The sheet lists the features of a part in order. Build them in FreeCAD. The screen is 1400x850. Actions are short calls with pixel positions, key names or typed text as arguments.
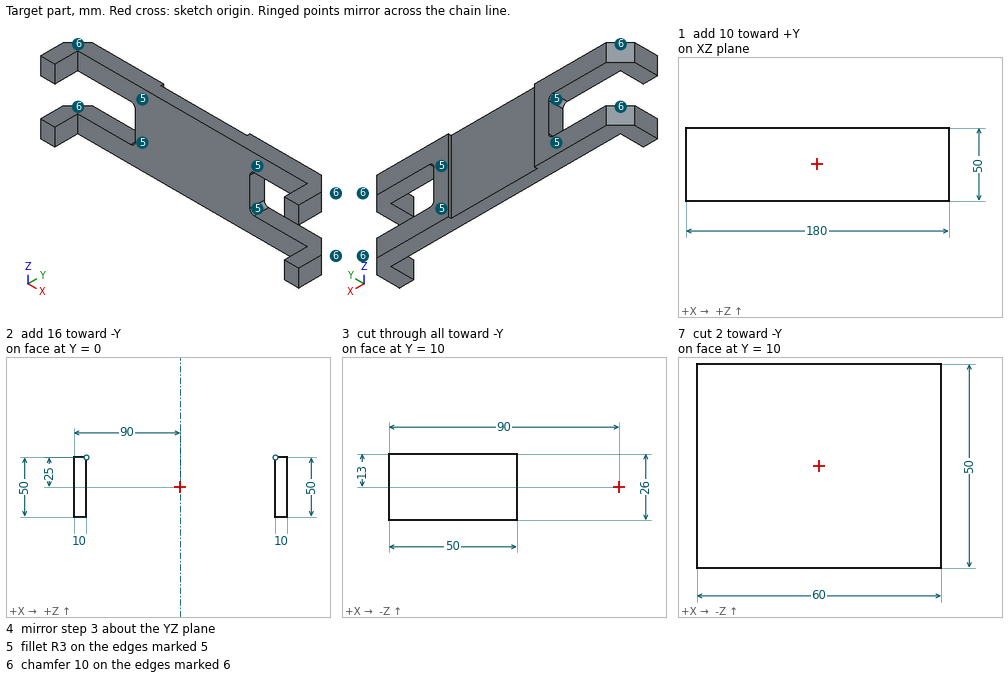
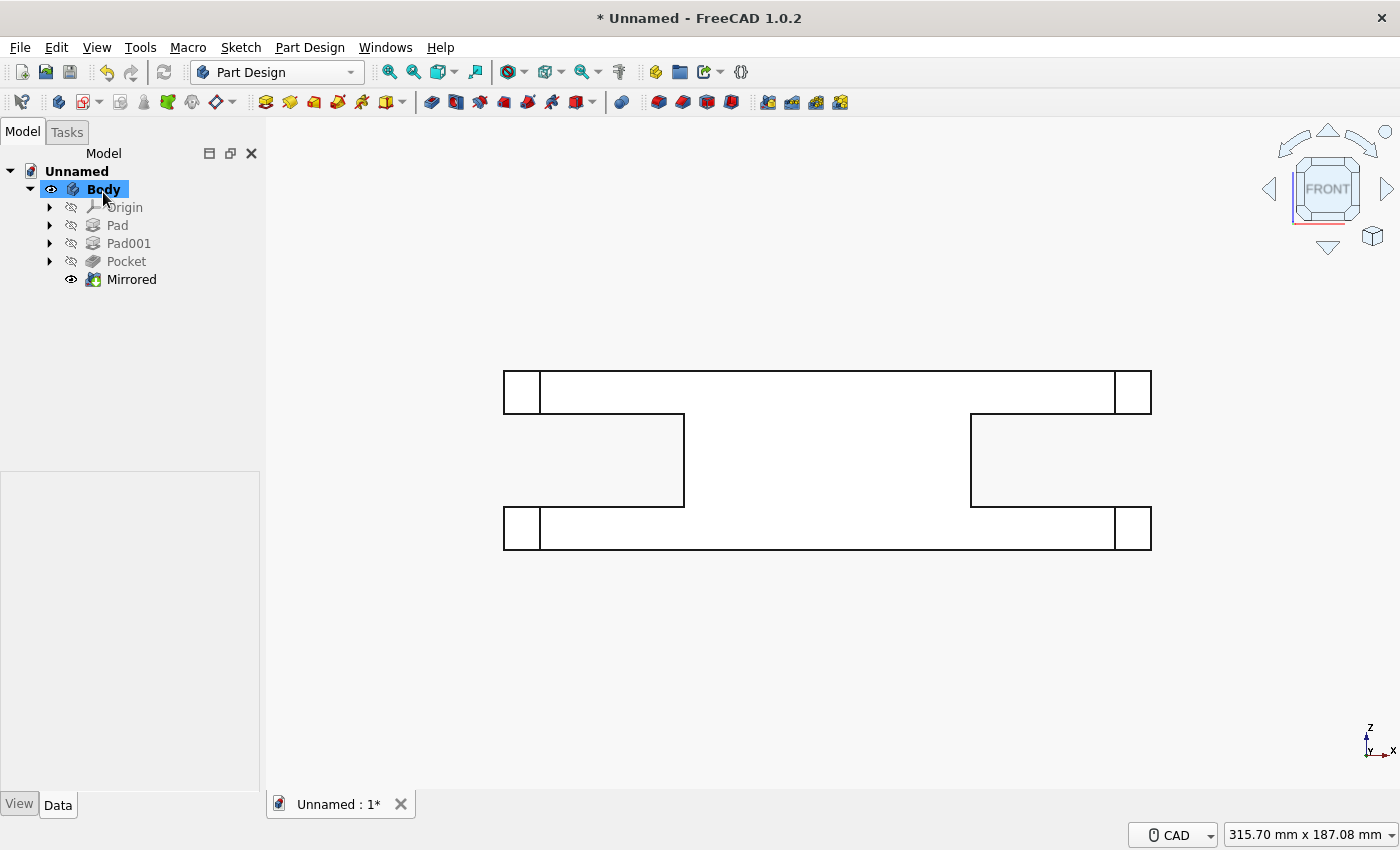
key(3)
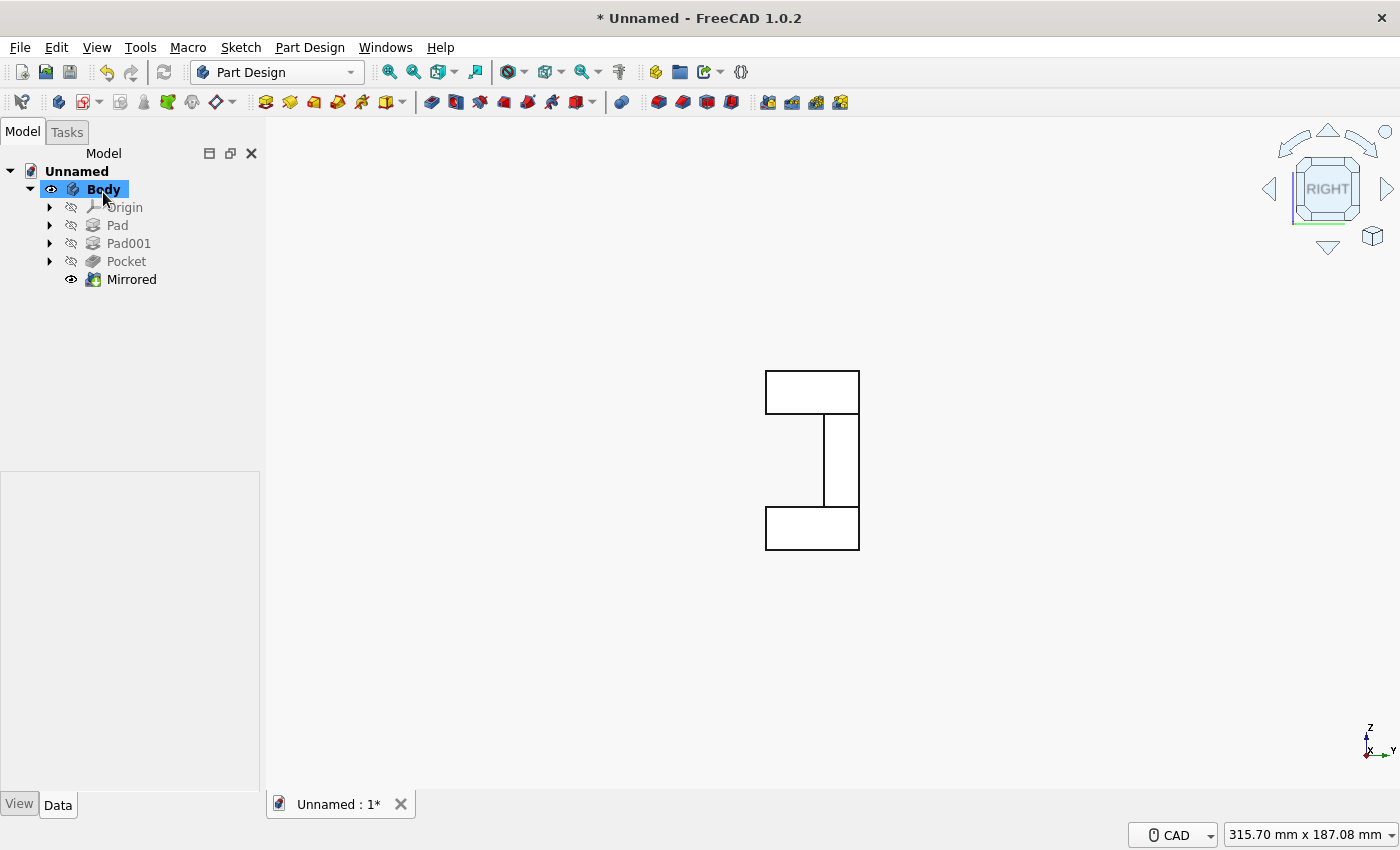
click(390, 72)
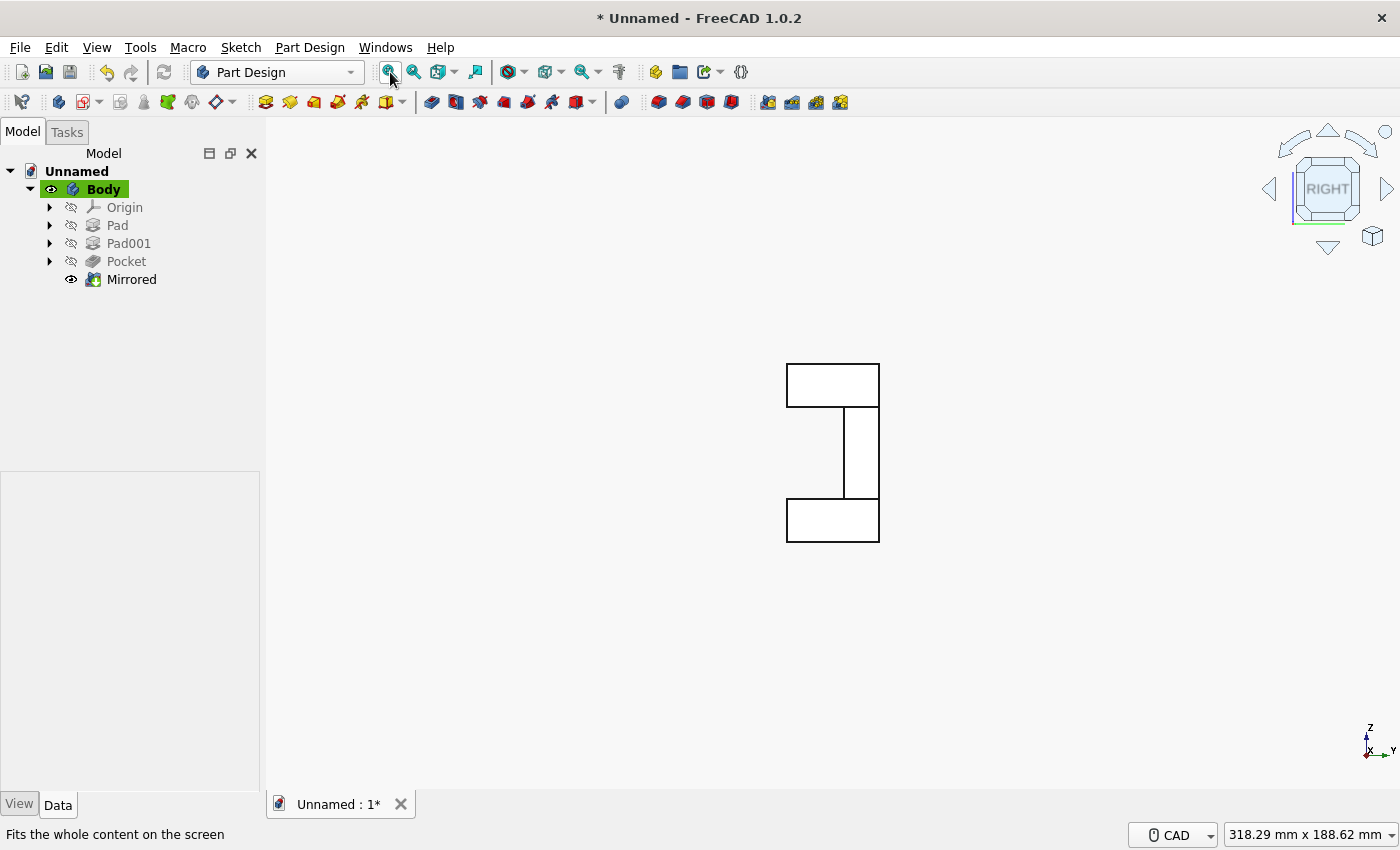
key(5)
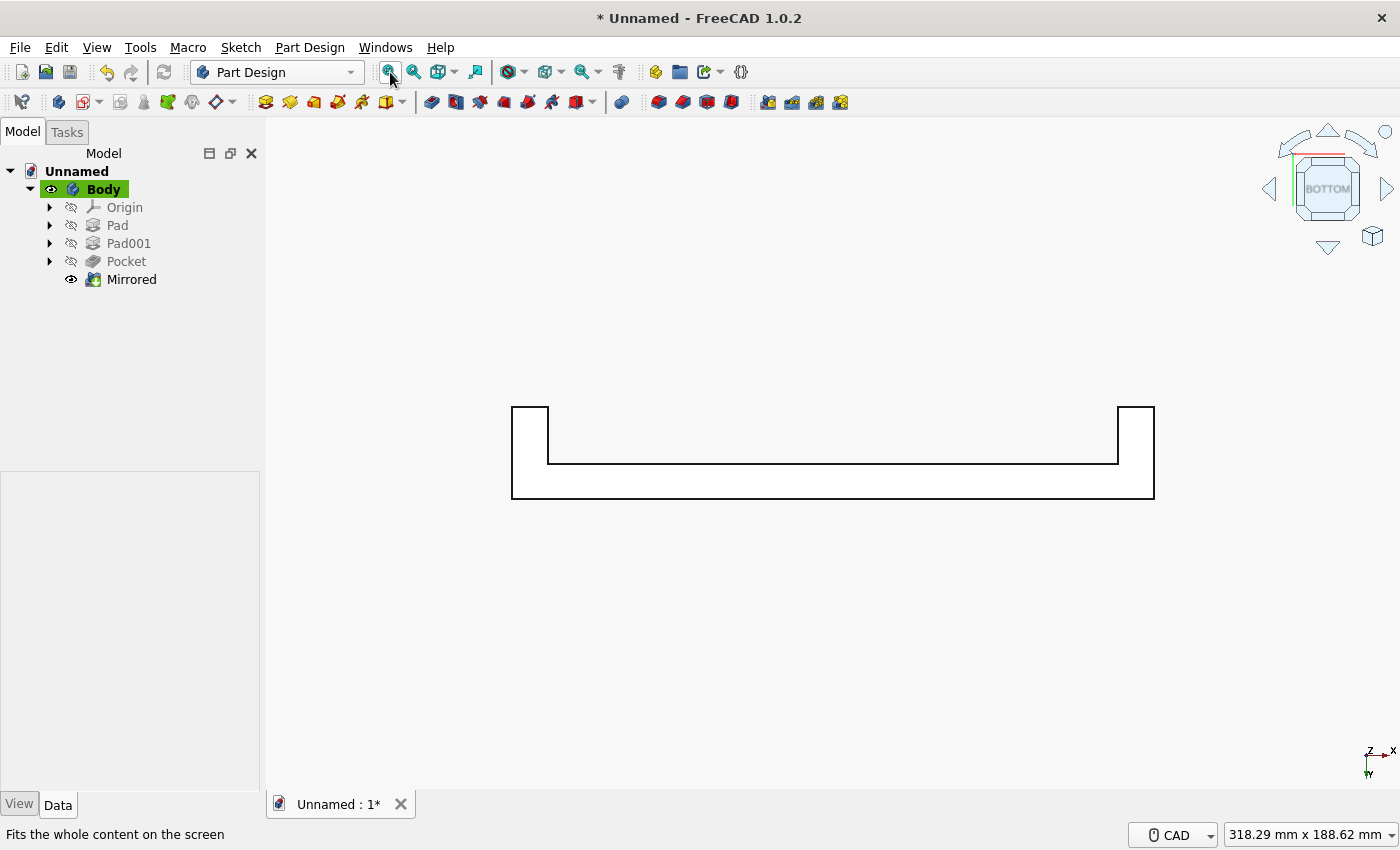
key(4)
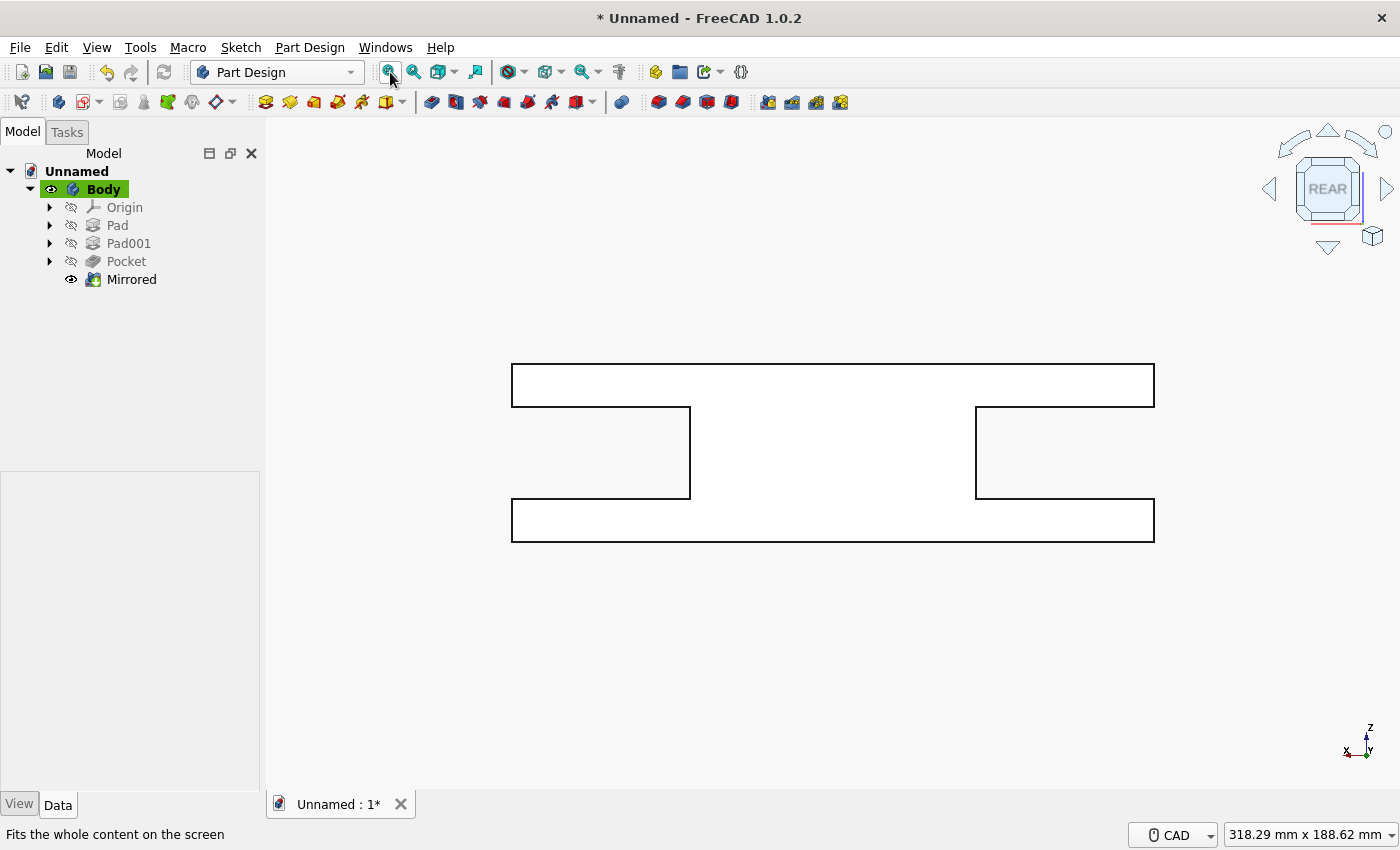
key(6)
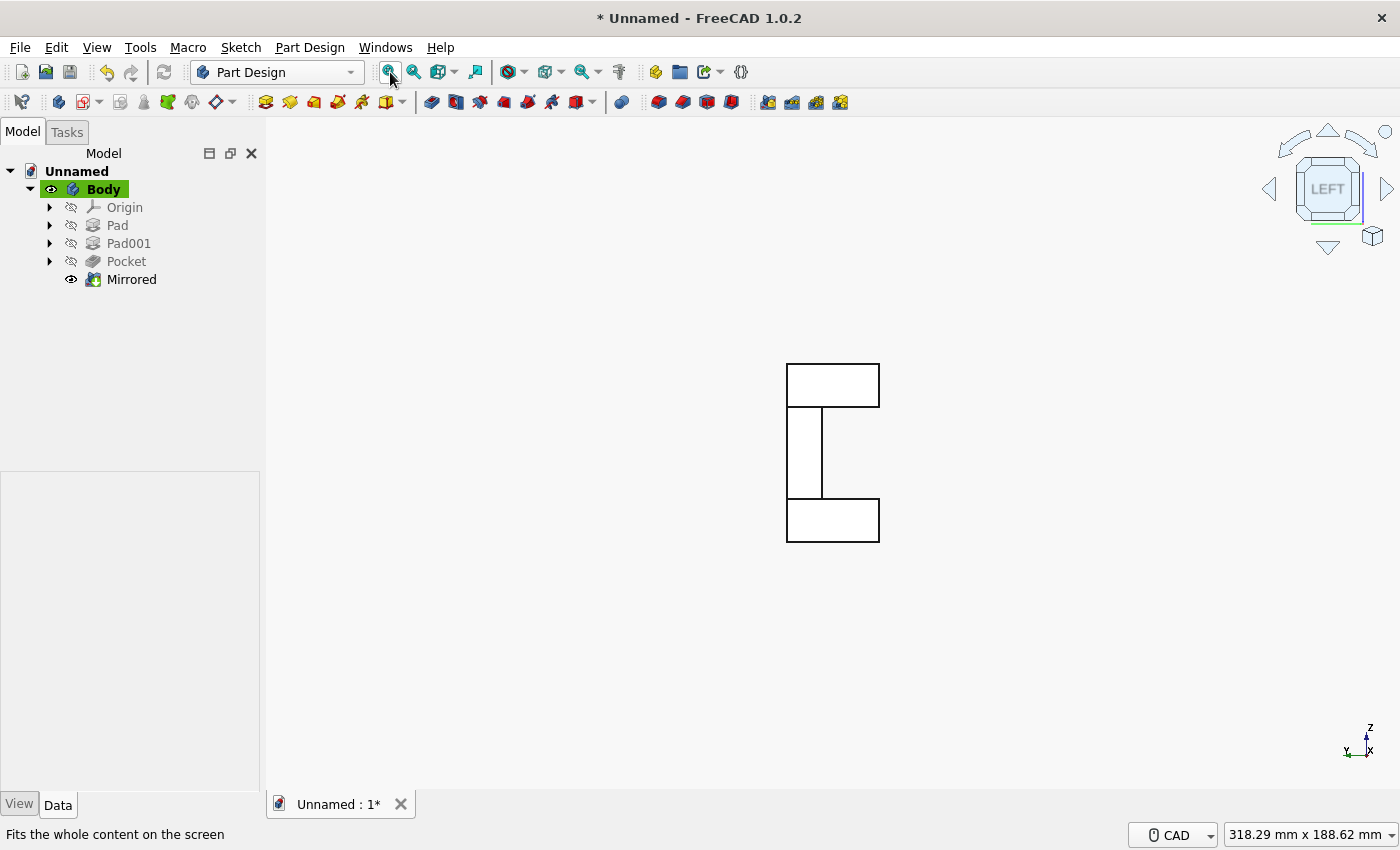
key(v)
key(f)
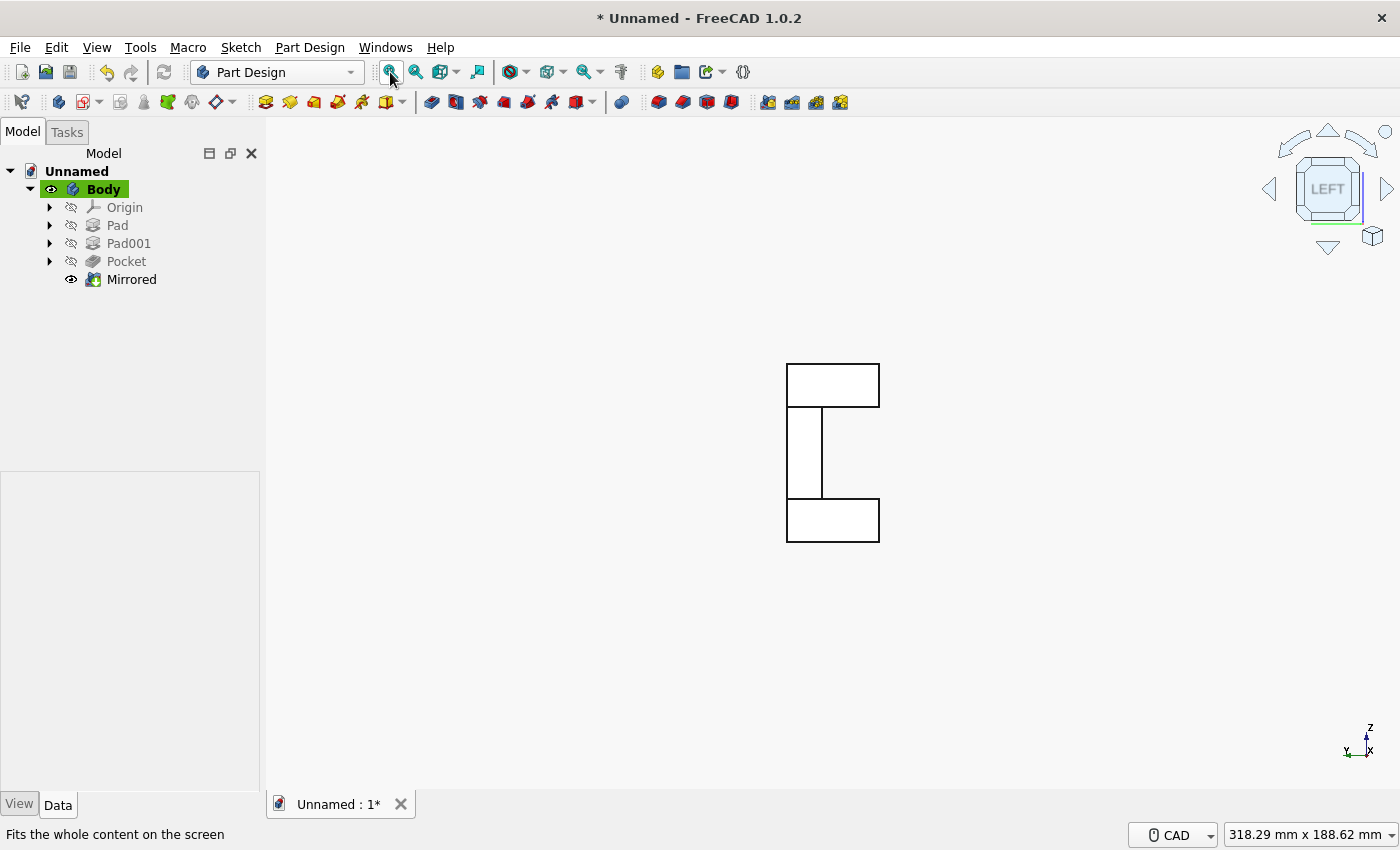
key(v)
key(3)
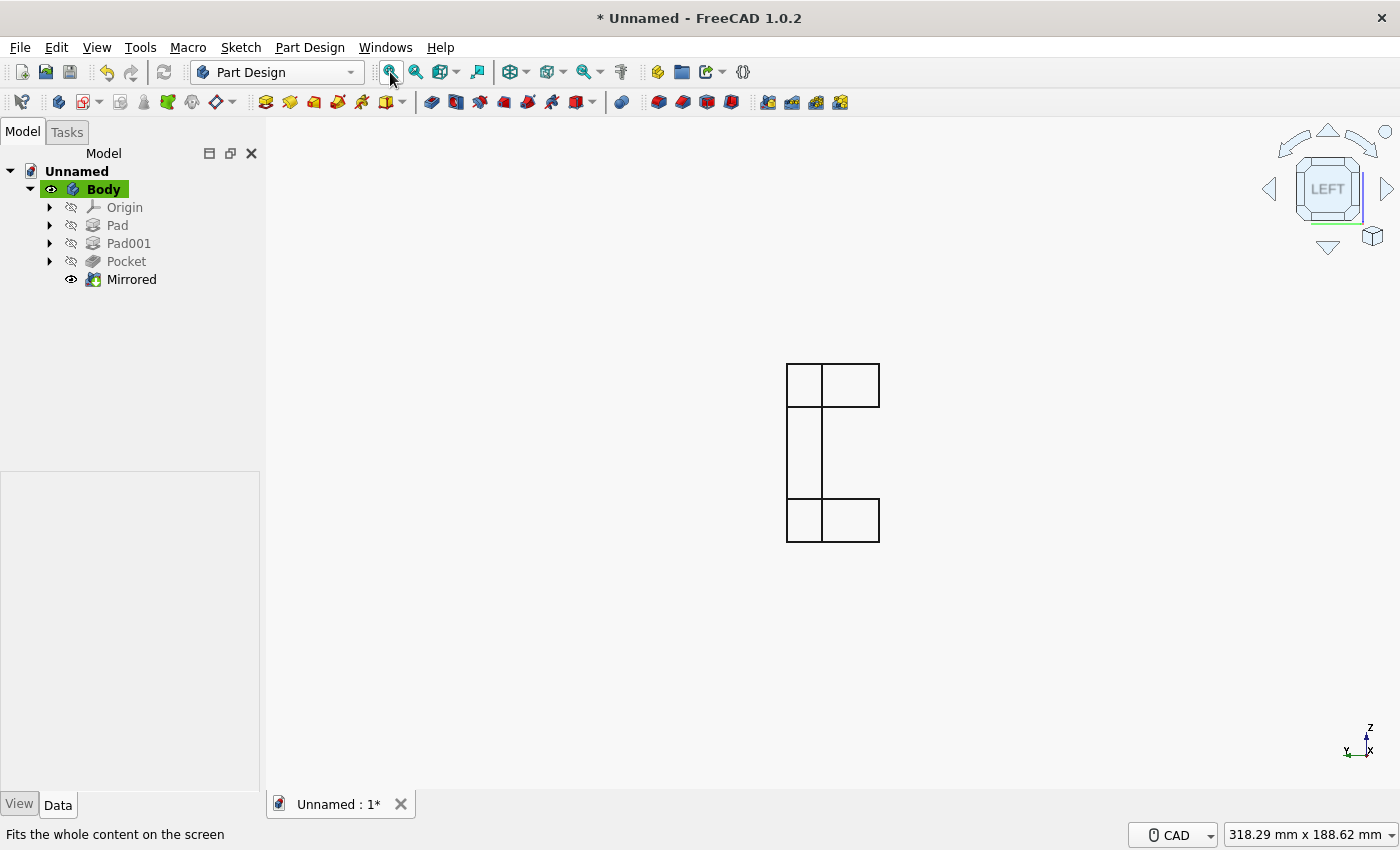
key(0)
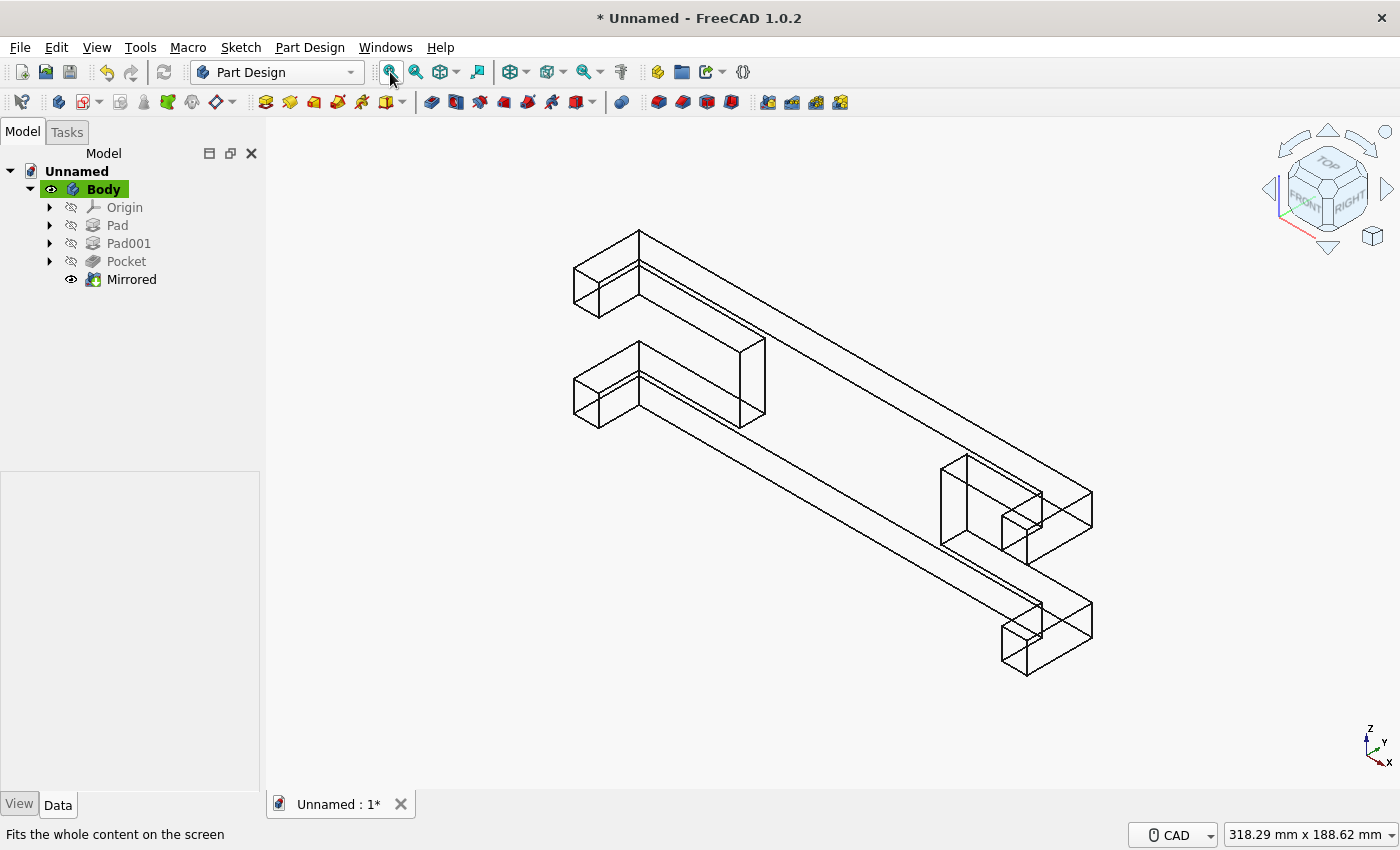
click(752, 420)